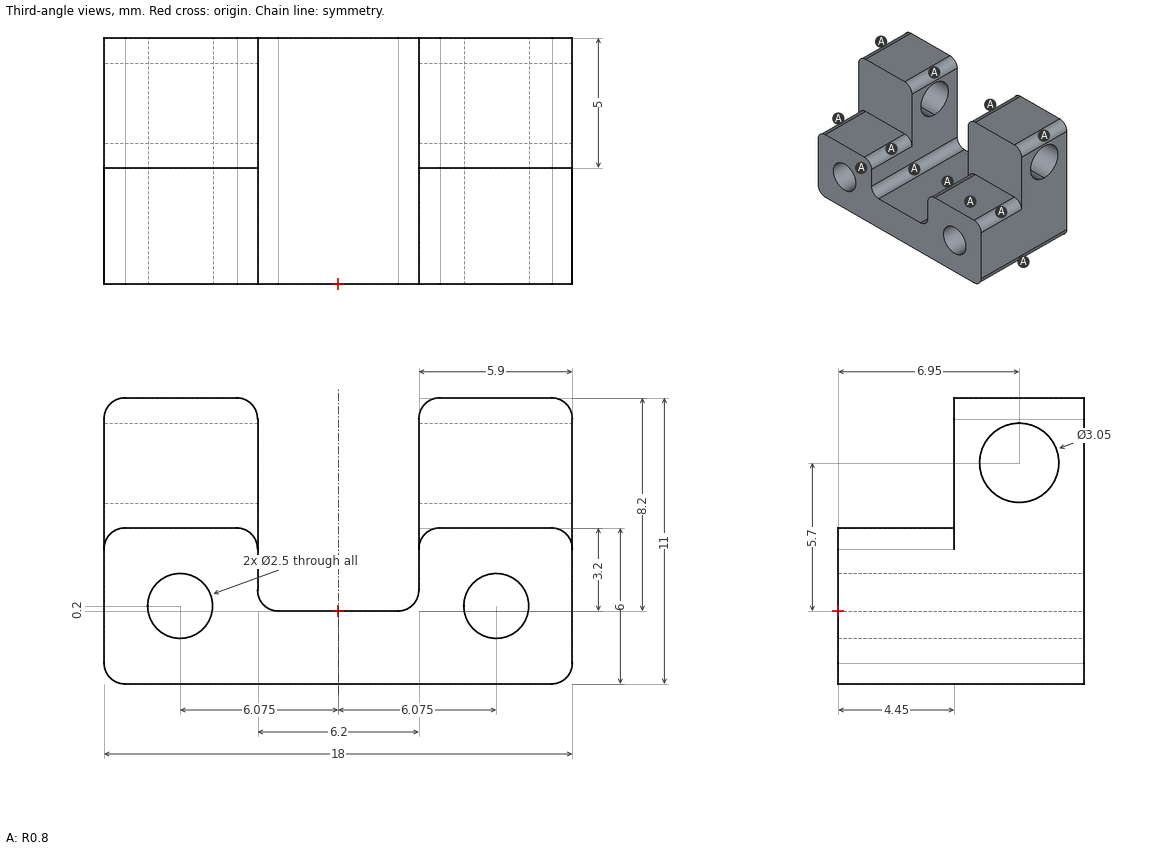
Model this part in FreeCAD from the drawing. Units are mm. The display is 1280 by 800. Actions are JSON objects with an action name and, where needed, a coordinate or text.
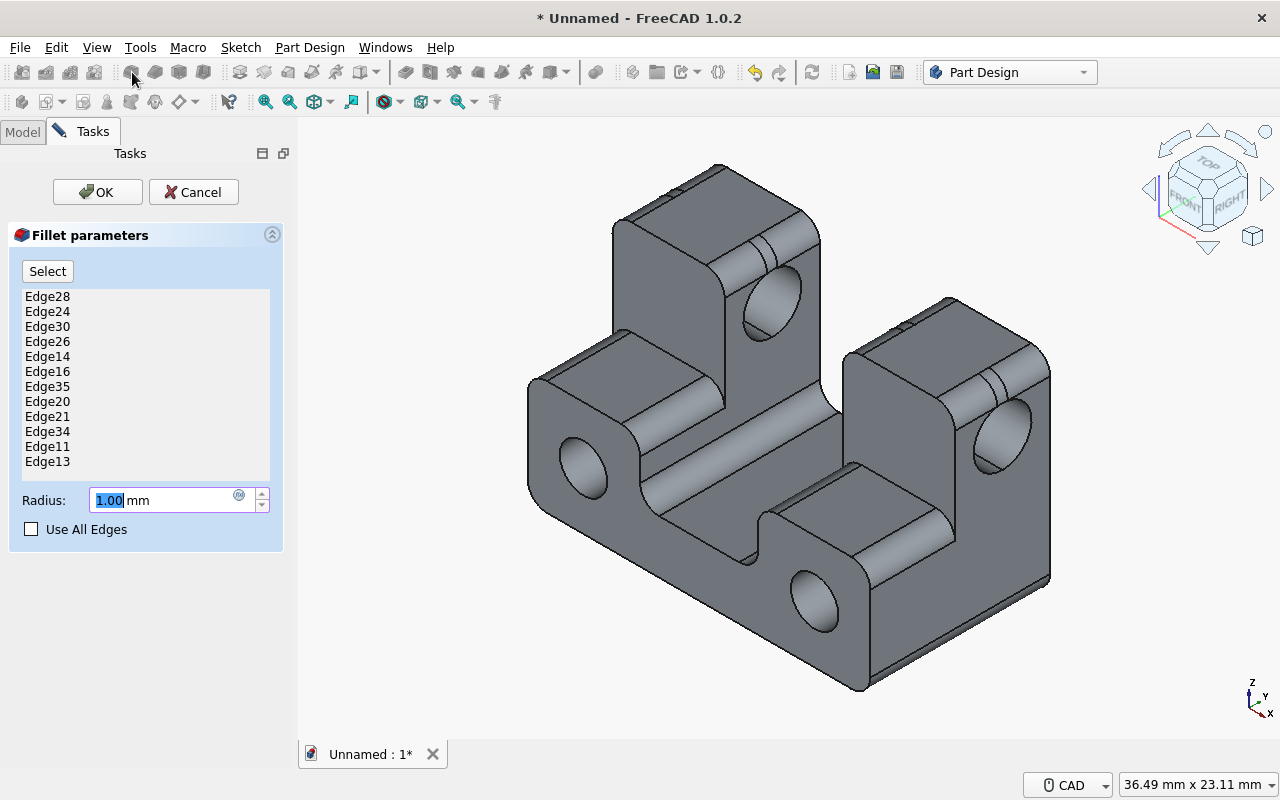
{"action": "type", "text": "0.8"}
{"action": "key", "text": "Tab"}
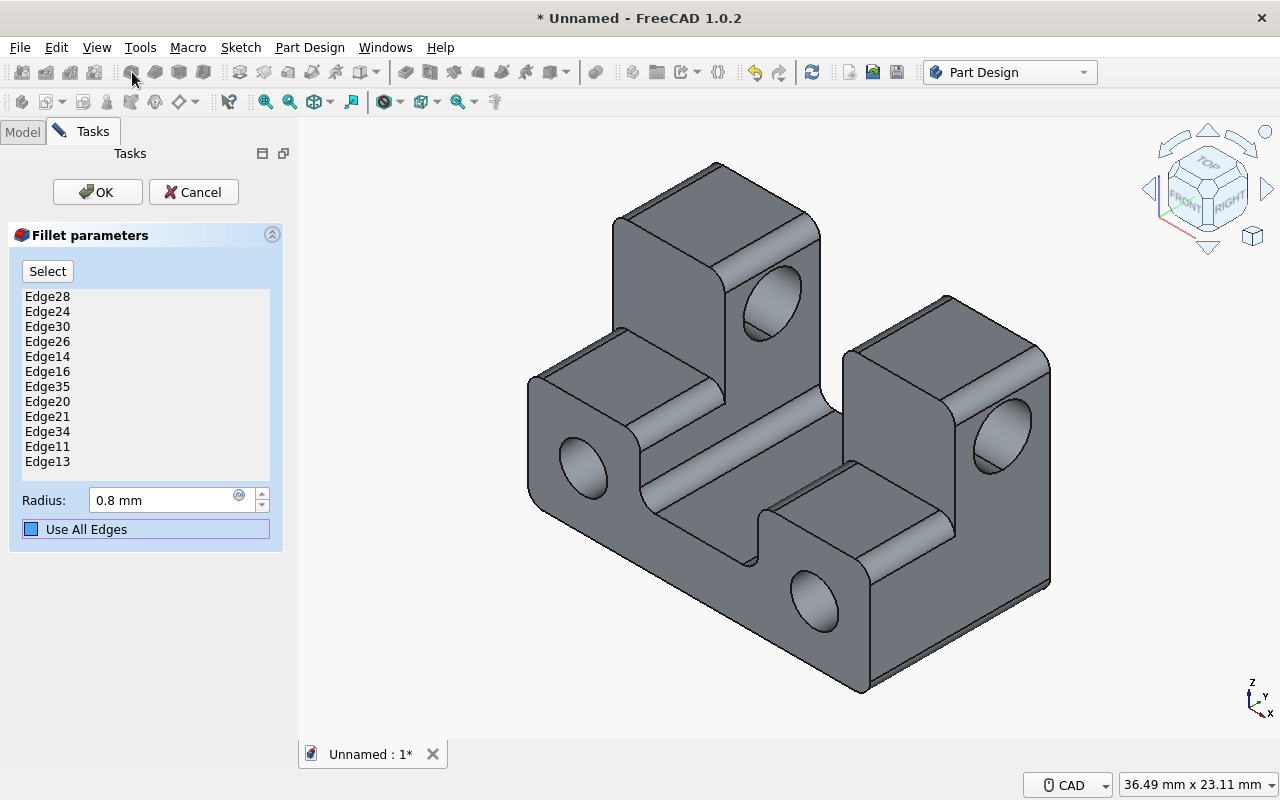
{"action": "left_click", "coordinate": [98, 192]}